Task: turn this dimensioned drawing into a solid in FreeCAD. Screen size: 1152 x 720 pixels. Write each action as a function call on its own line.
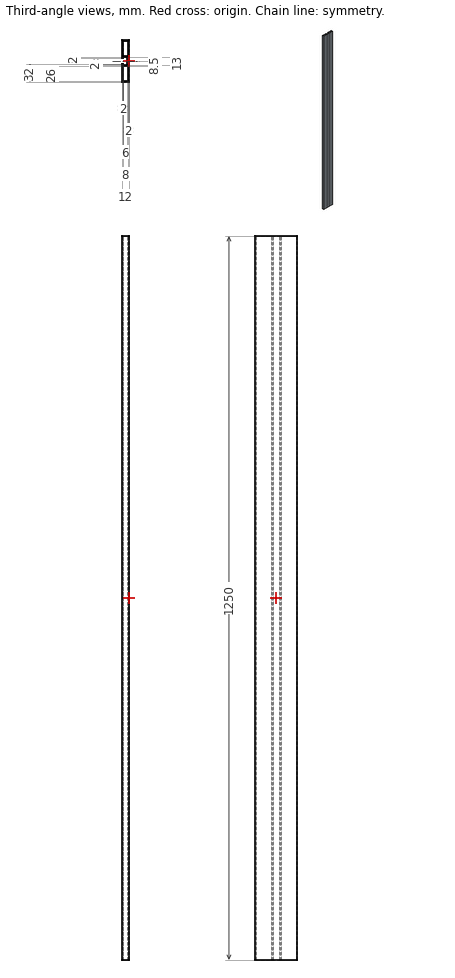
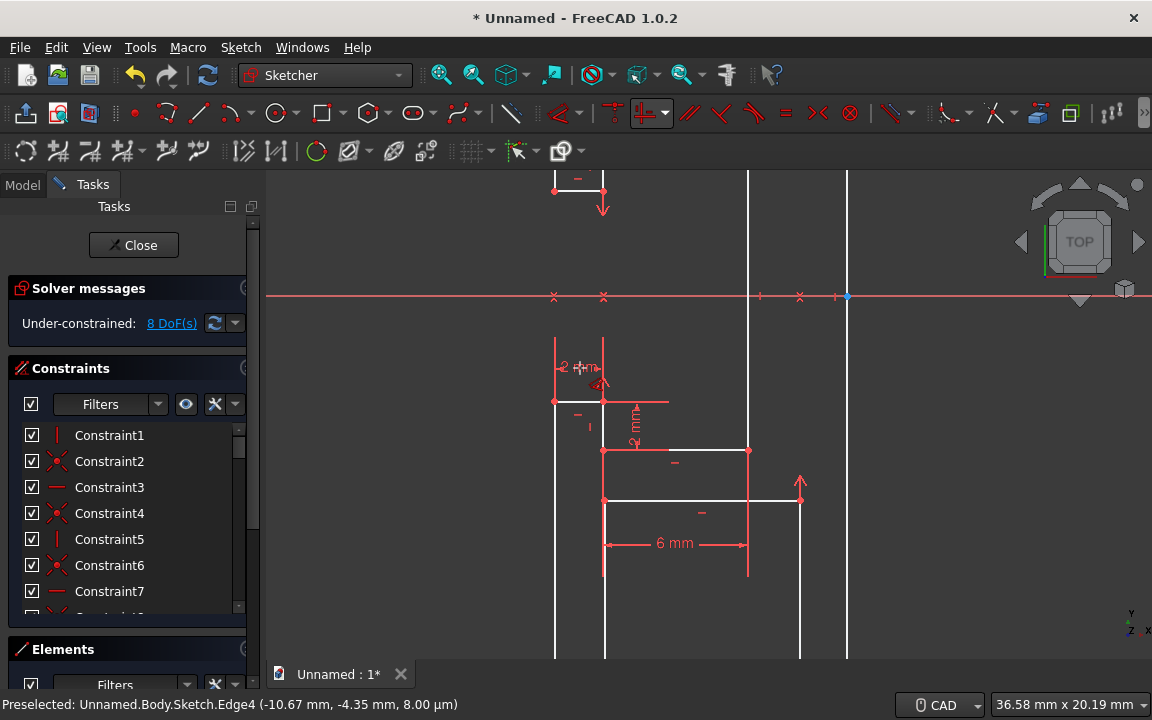
scroll(628, 438, down, 9)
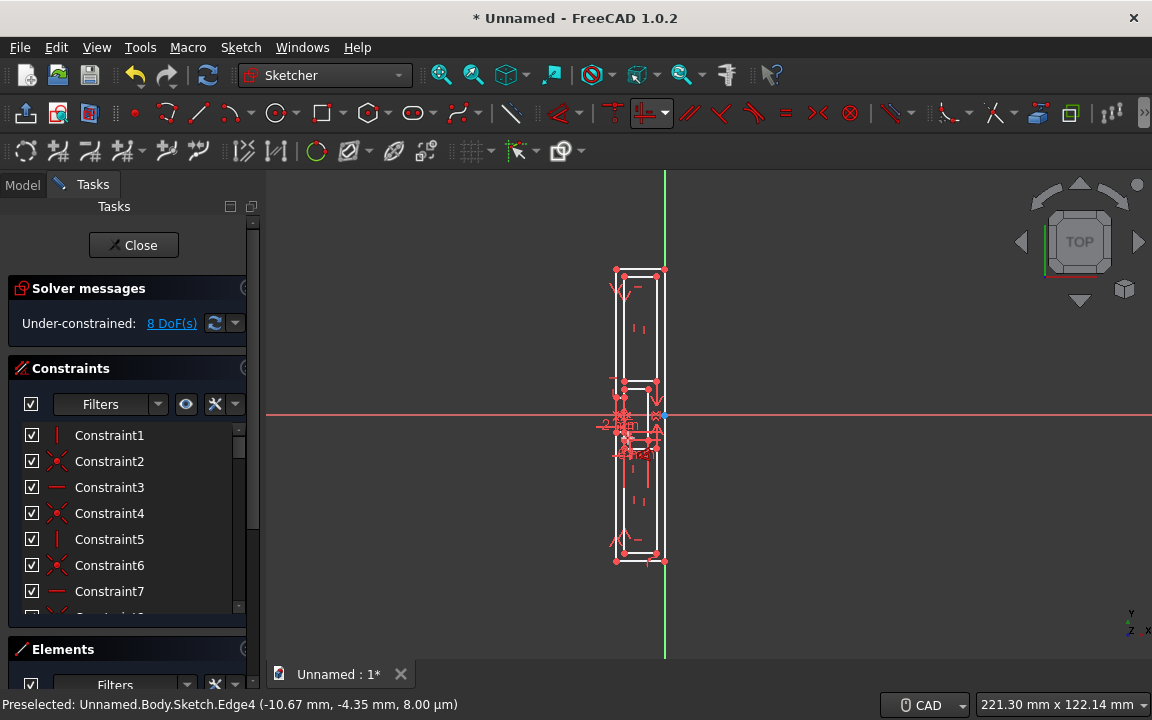
scroll(624, 395, up, 9)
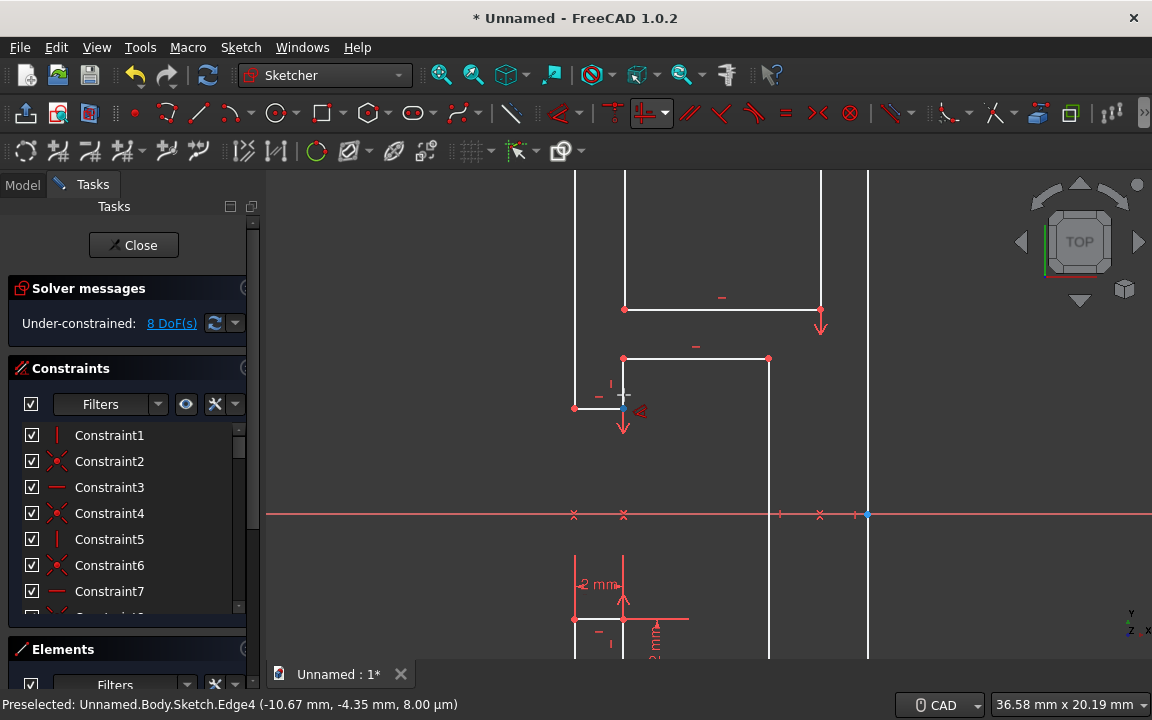
click(623, 394)
click(589, 384)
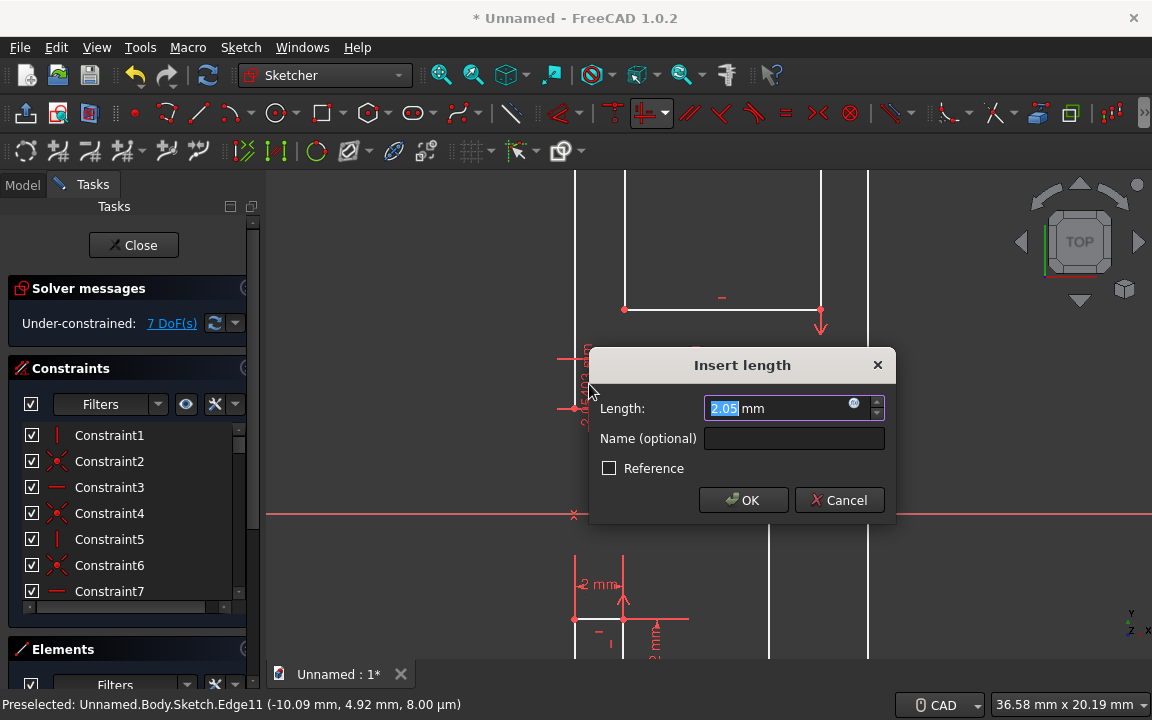
text(2)
key(Return)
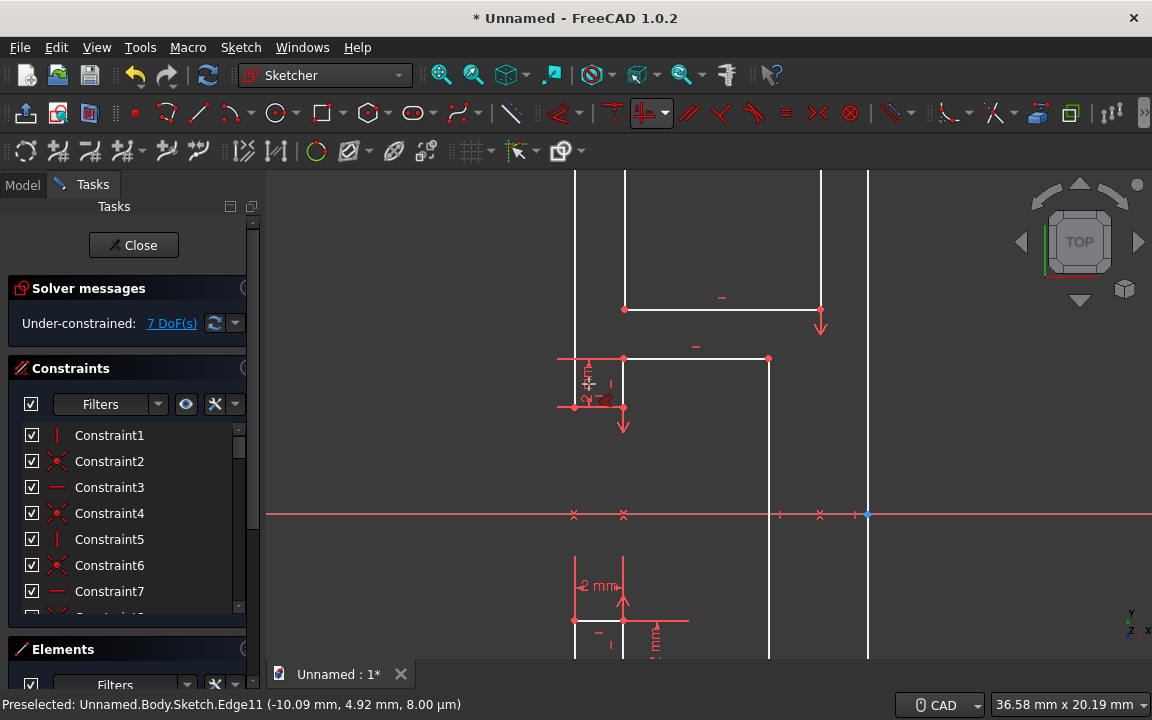
scroll(624, 395, down, 9)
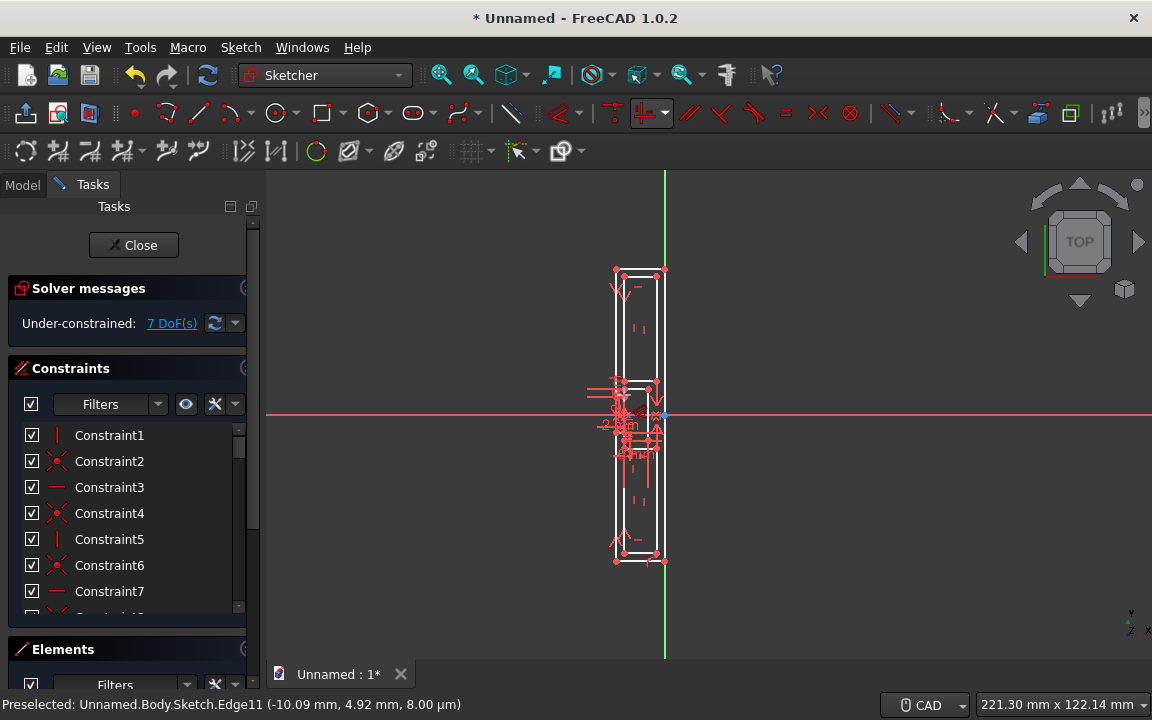
scroll(634, 553, up, 3)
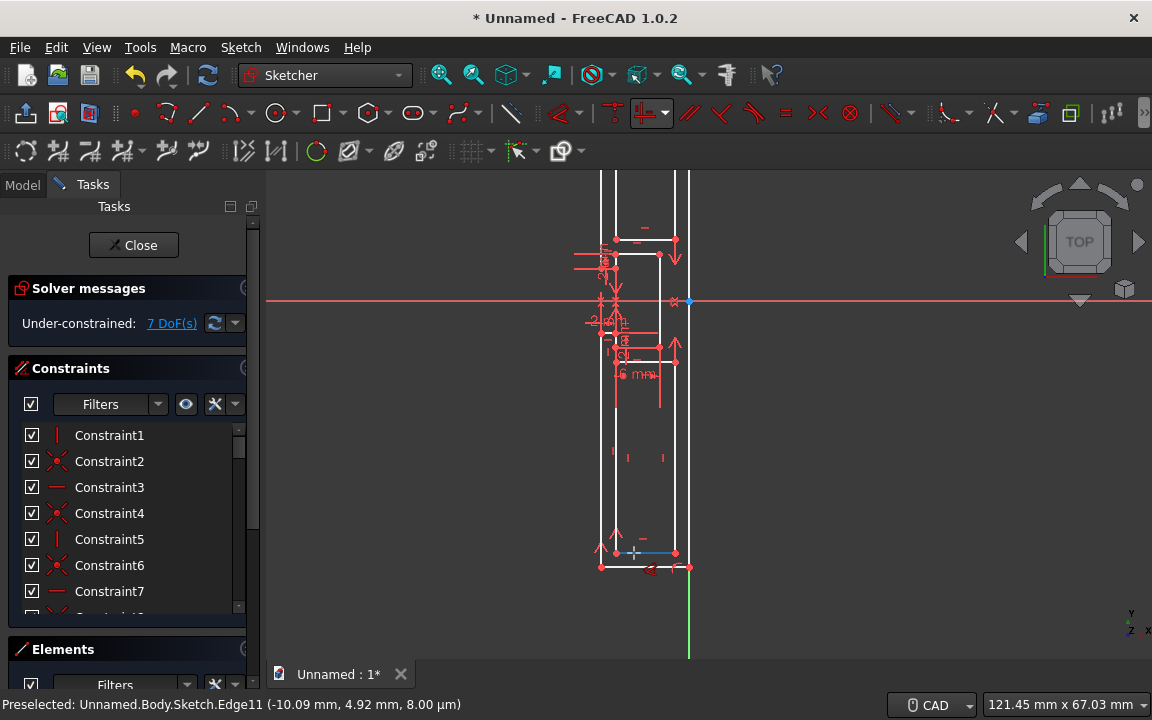
click(634, 553)
click(646, 587)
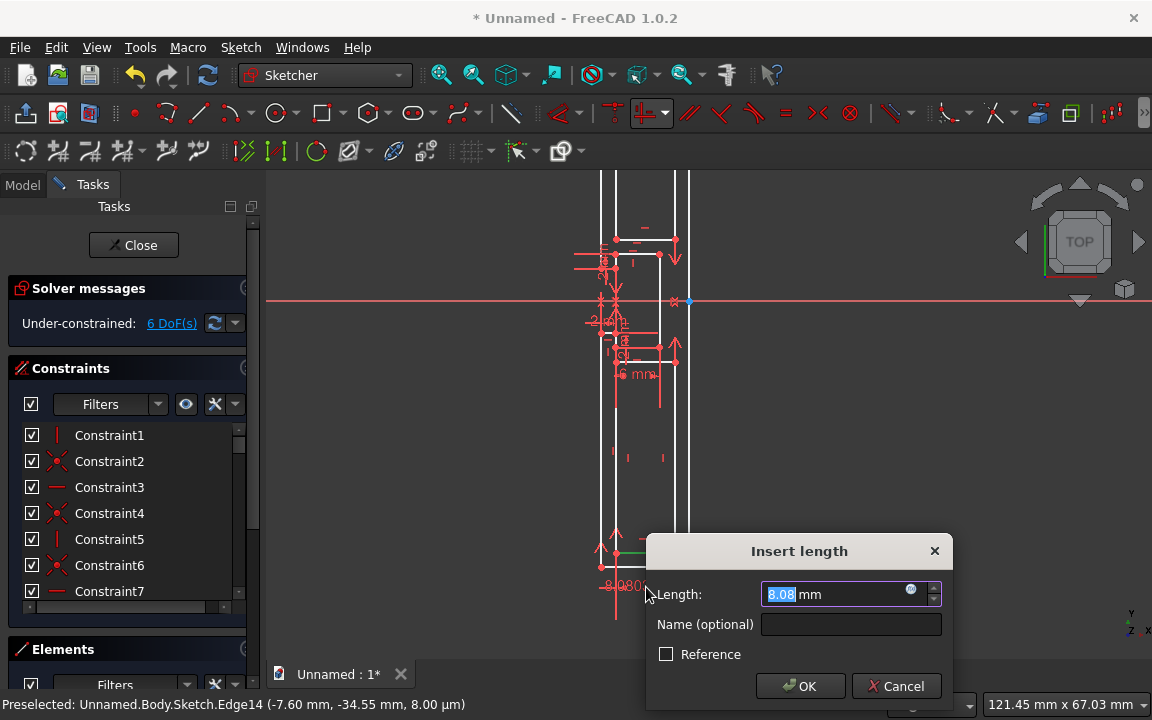
text(8)
key(Return)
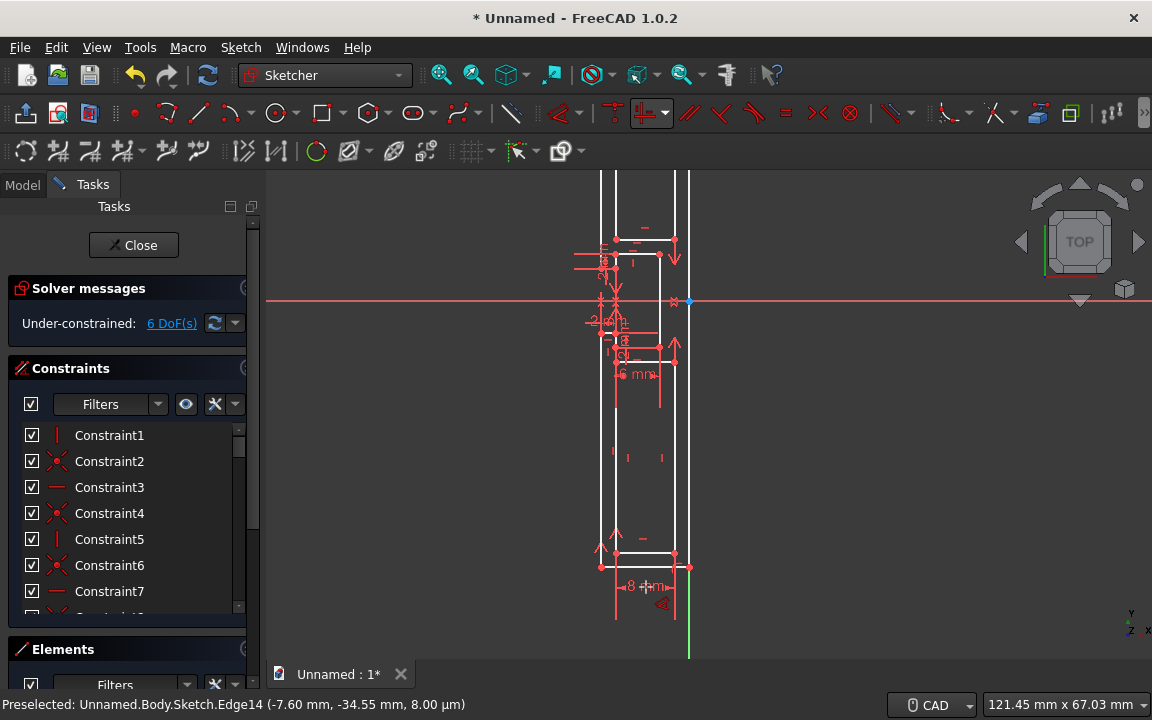
click(660, 282)
click(718, 280)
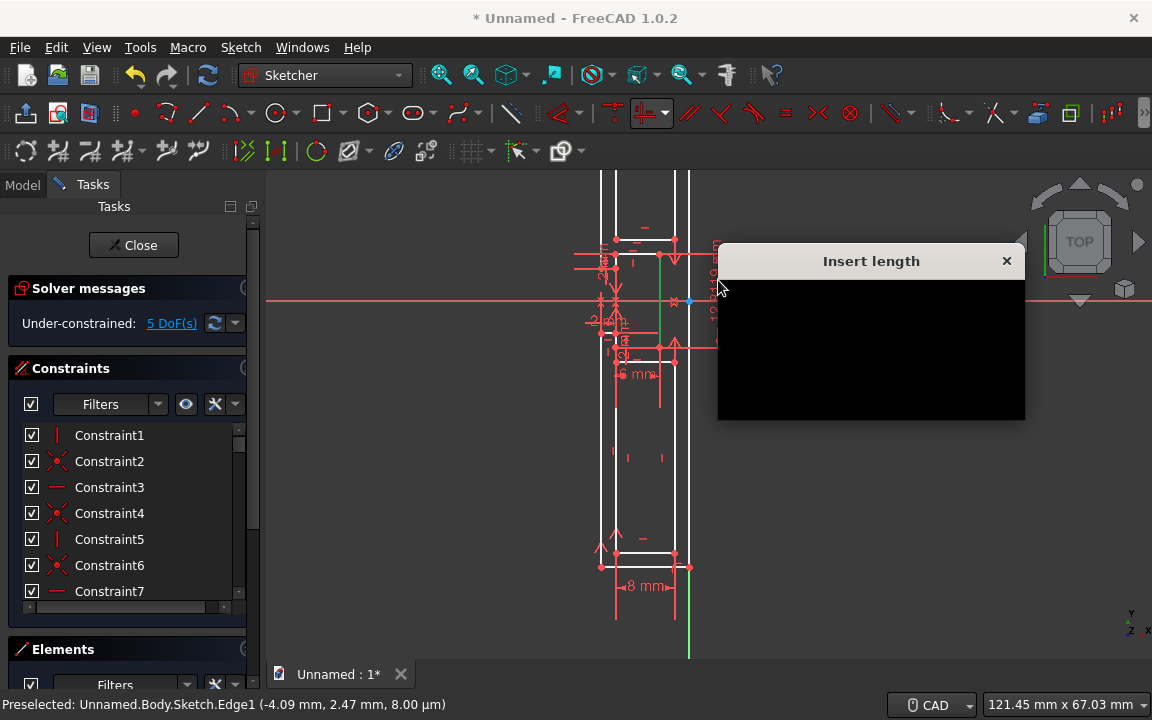
text(13)
key(Return)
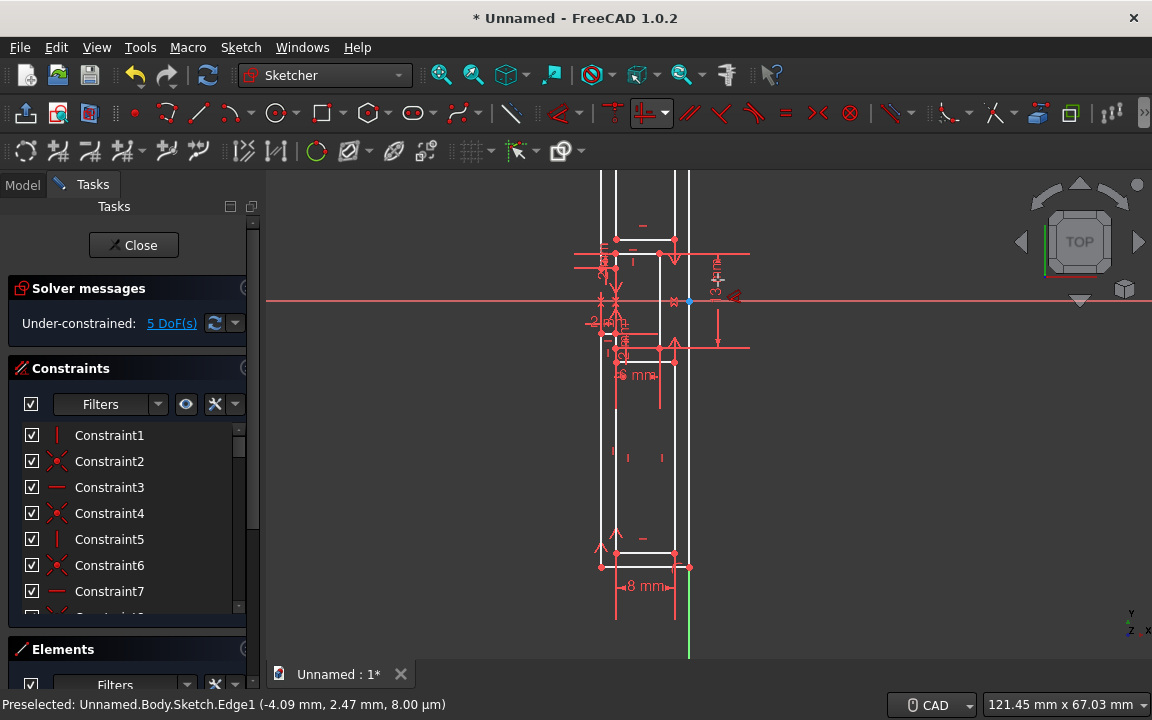
click(601, 404)
click(567, 450)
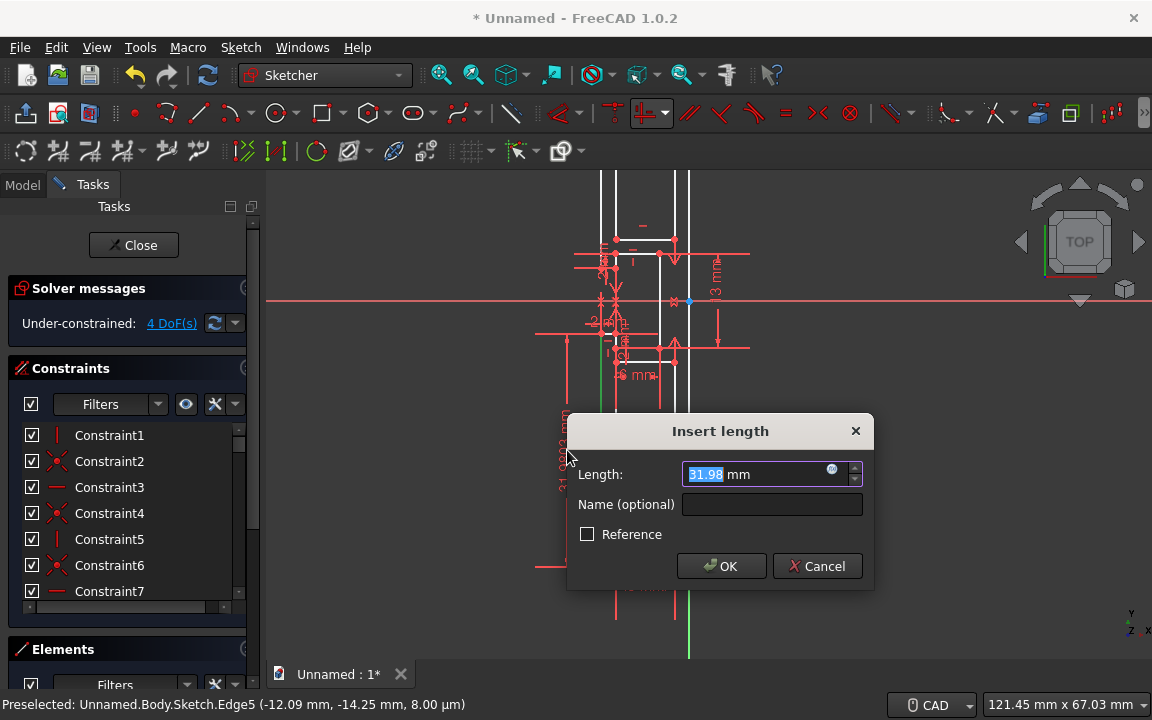
text(32)
key(Return)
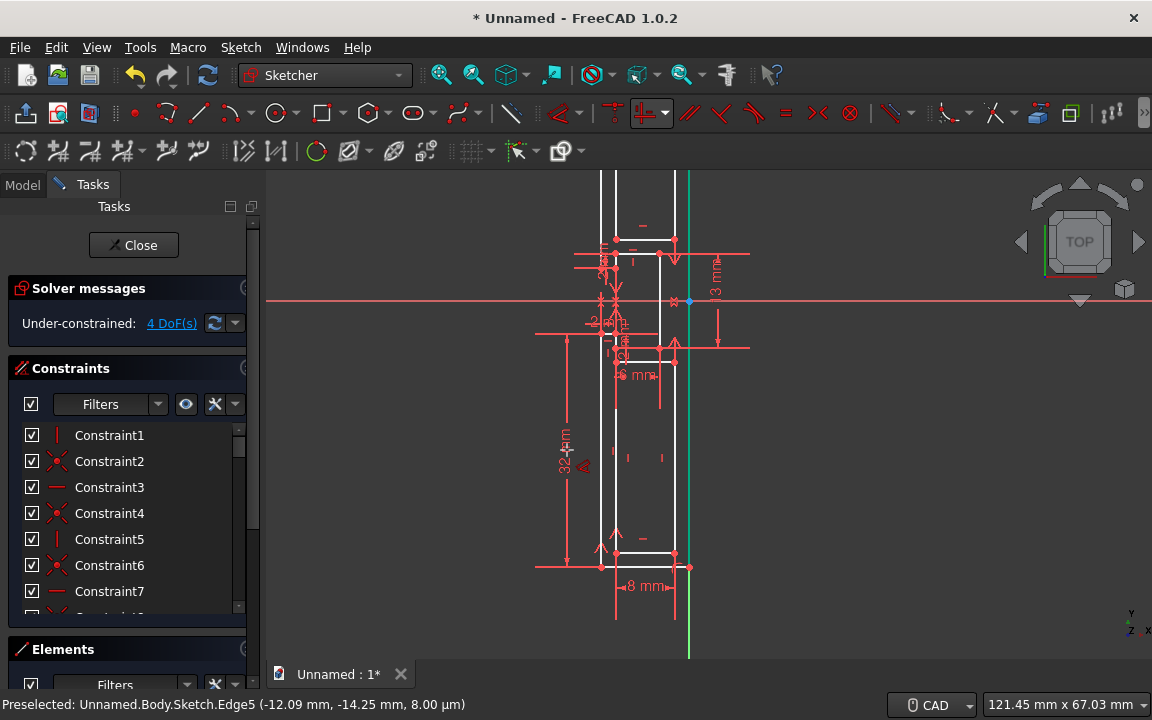
click(628, 567)
click(645, 533)